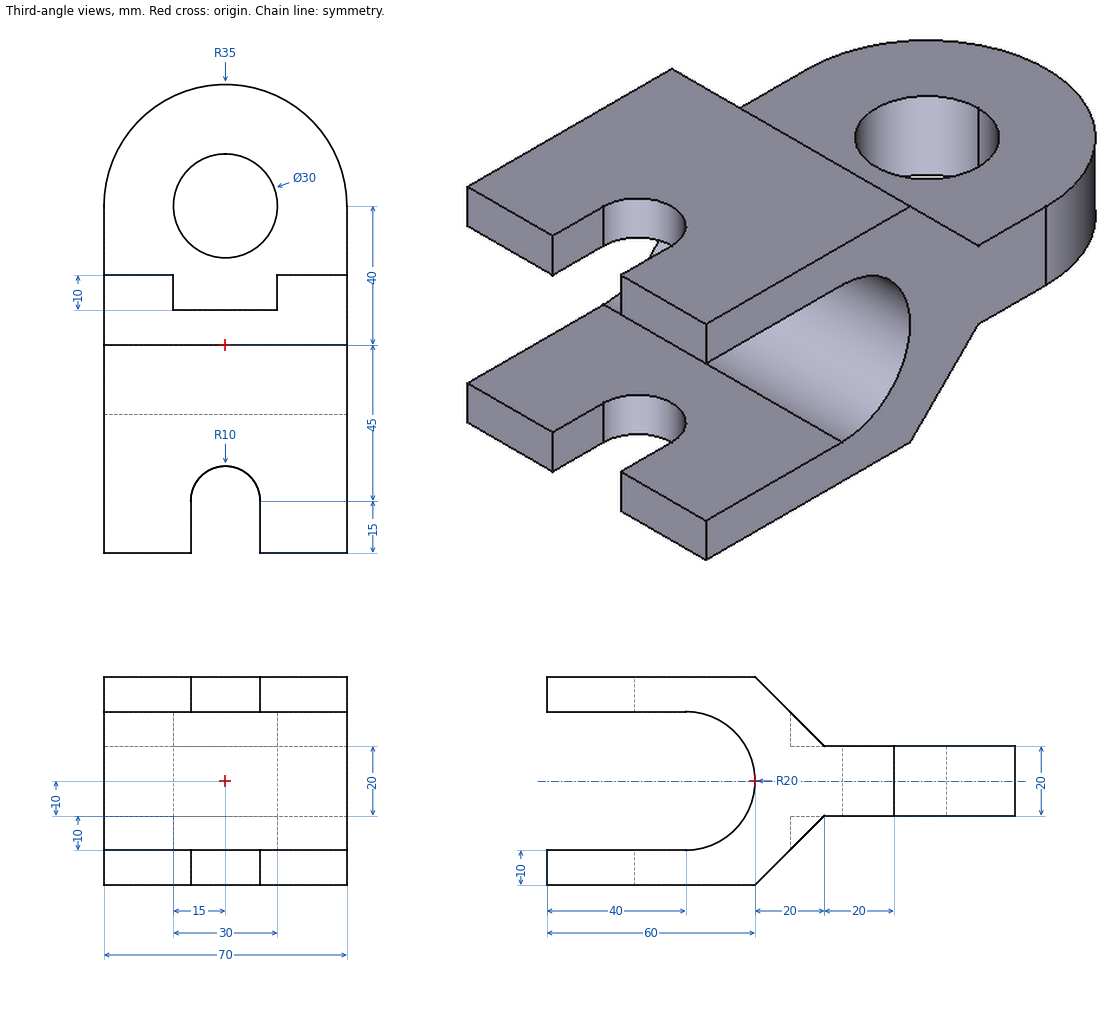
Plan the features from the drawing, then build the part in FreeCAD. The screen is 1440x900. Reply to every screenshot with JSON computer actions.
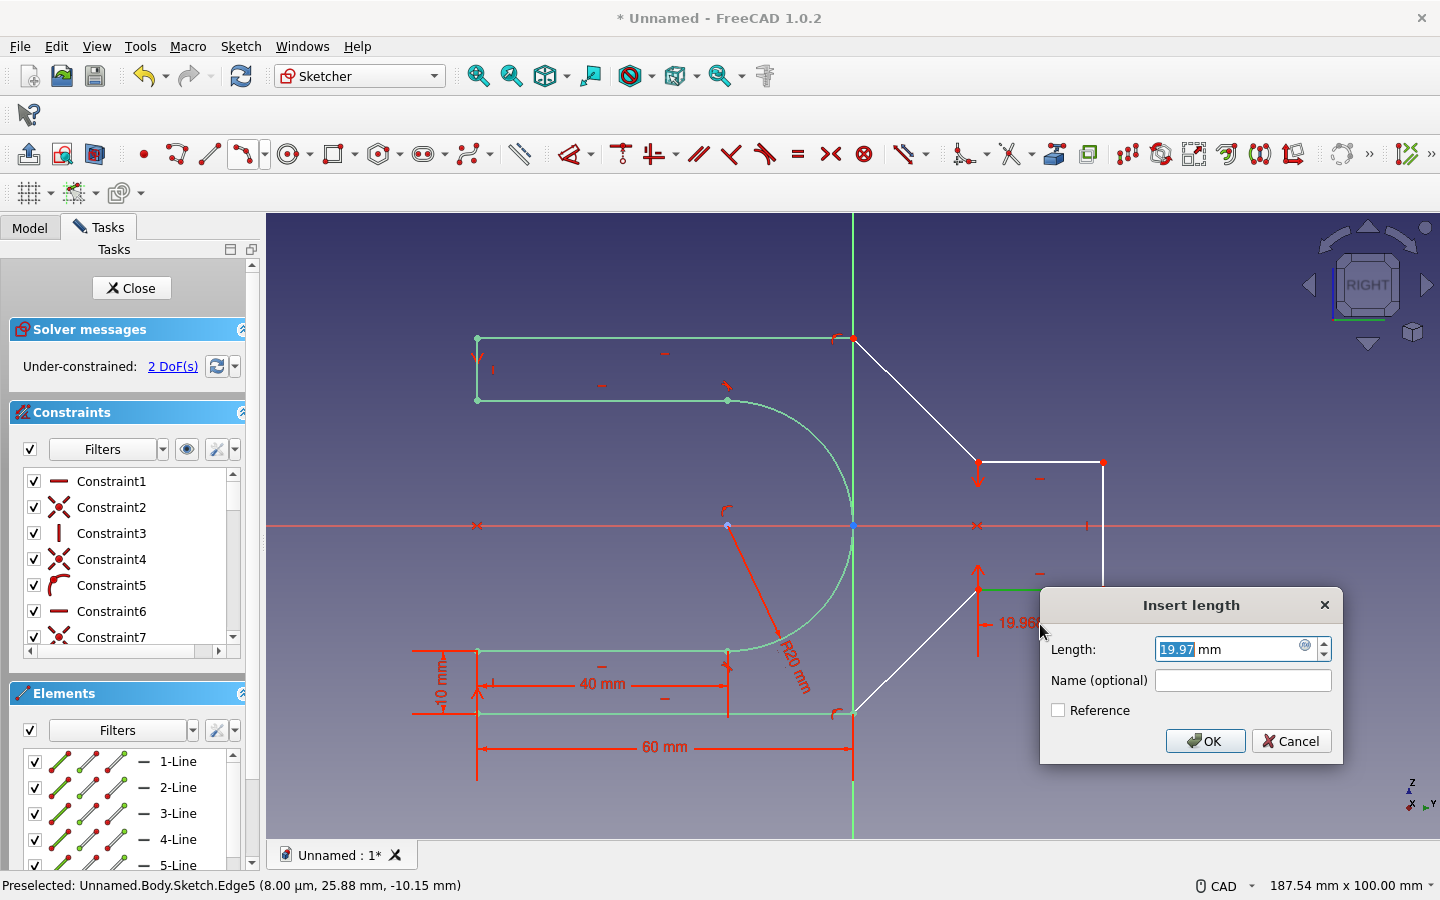
{"action": "type", "text": "20"}
{"action": "key", "text": "Return"}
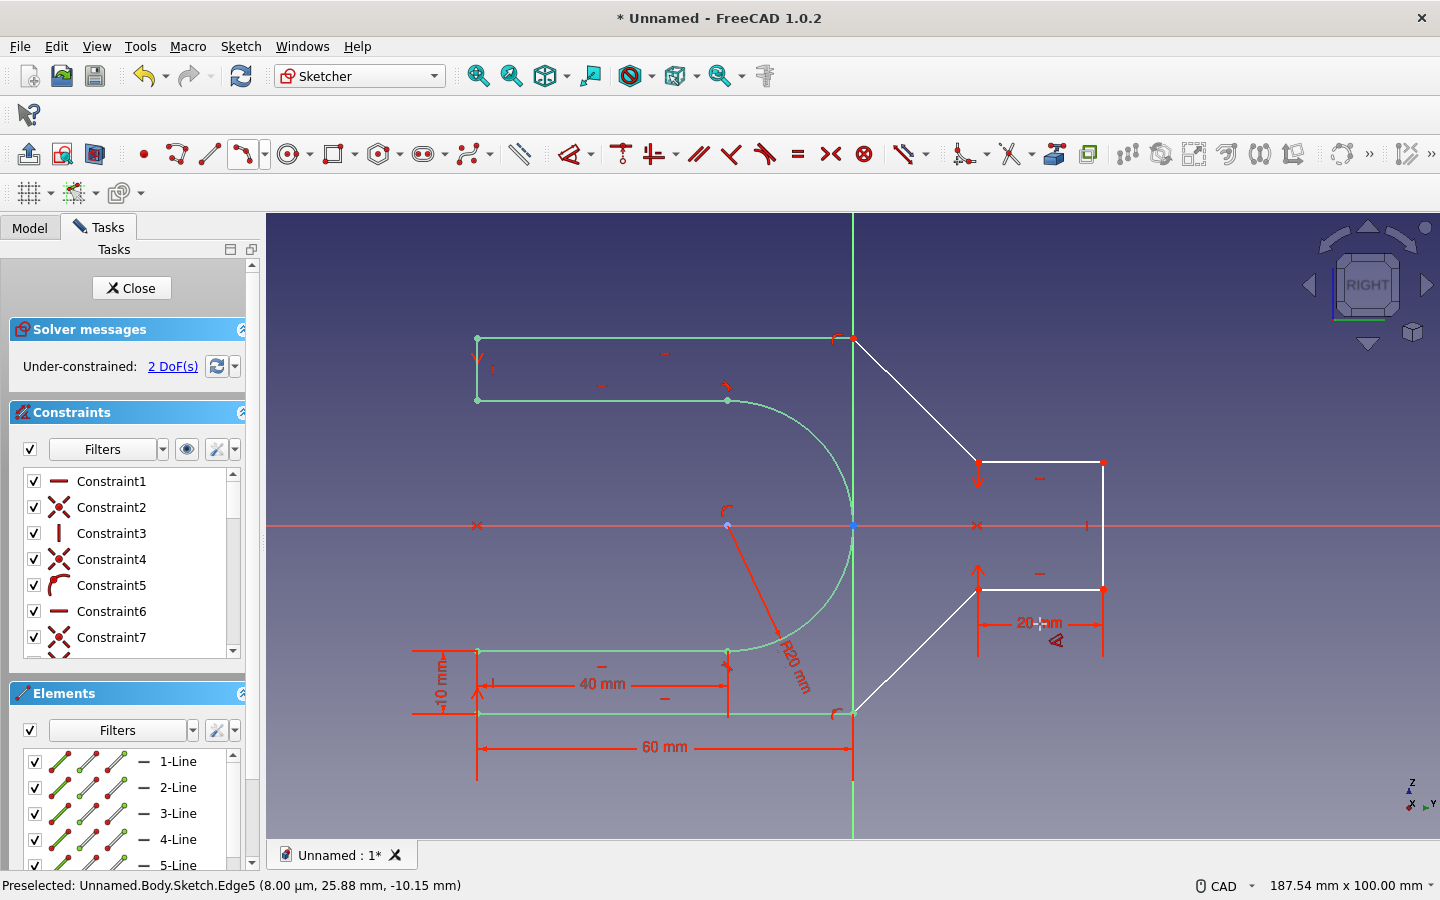
{"action": "left_click", "coordinate": [1103, 551]}
{"action": "left_click", "coordinate": [1137, 497]}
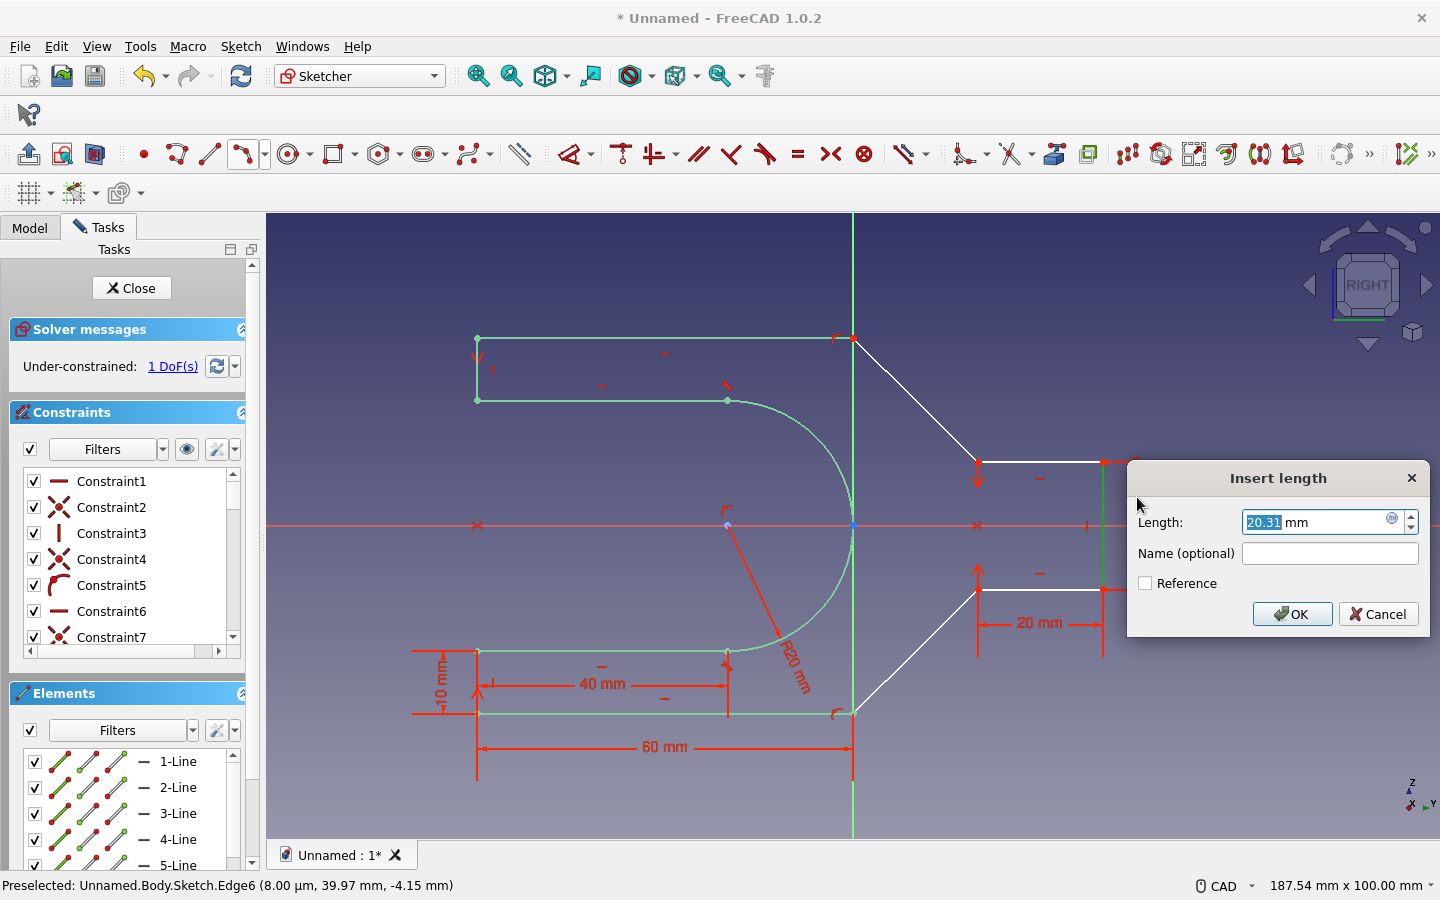
{"action": "type", "text": "20"}
{"action": "key", "text": "Return"}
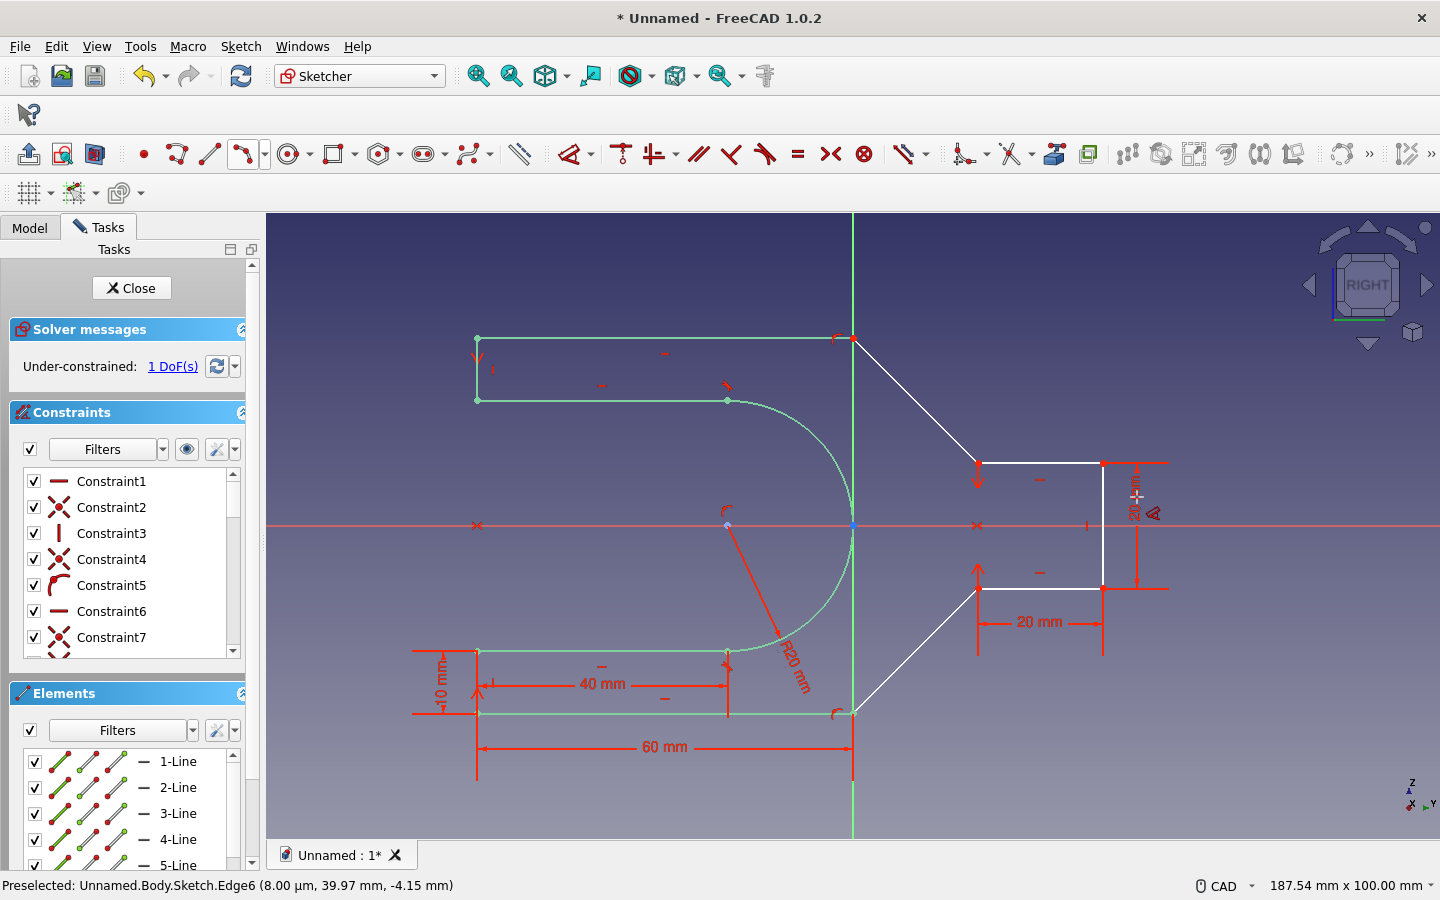
{"action": "left_click", "coordinate": [978, 589]}
{"action": "left_click", "coordinate": [915, 623]}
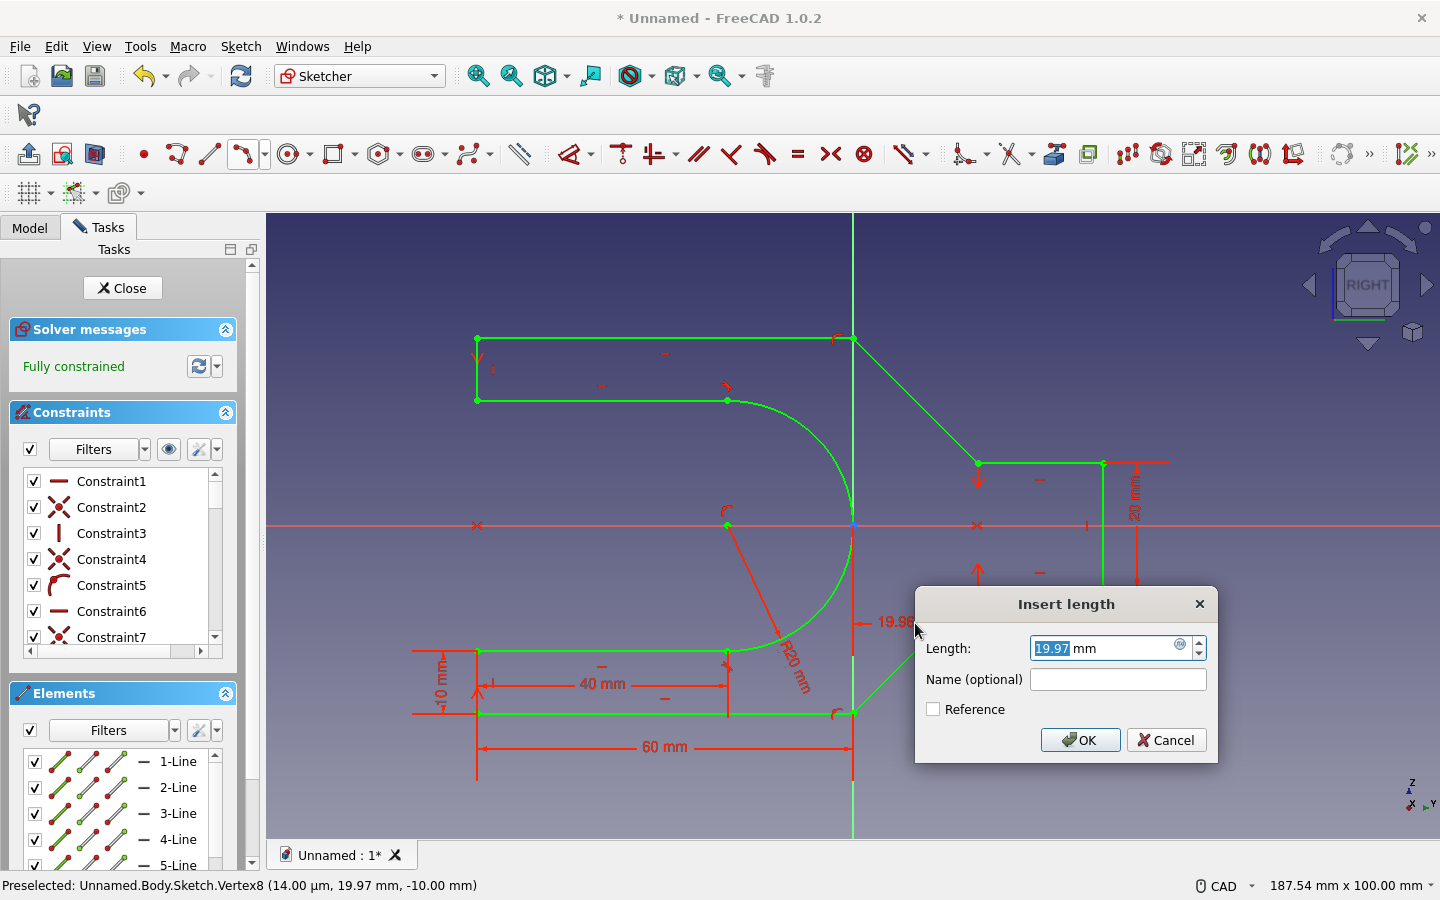
{"action": "type", "text": "20"}
{"action": "key", "text": "Return"}
{"action": "key", "text": "Escape"}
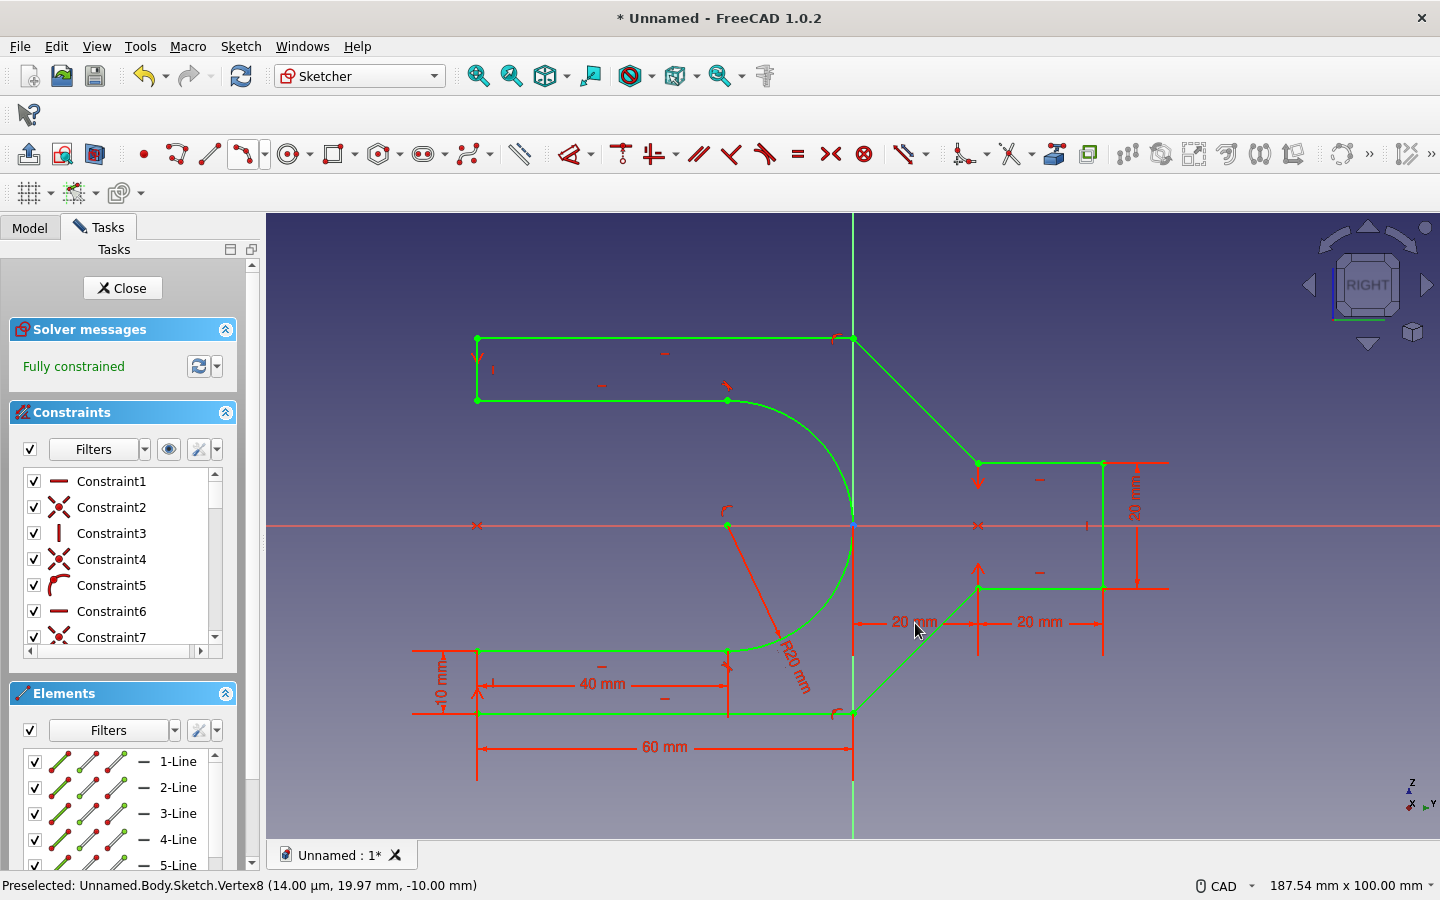
{"action": "left_click", "coordinate": [123, 288]}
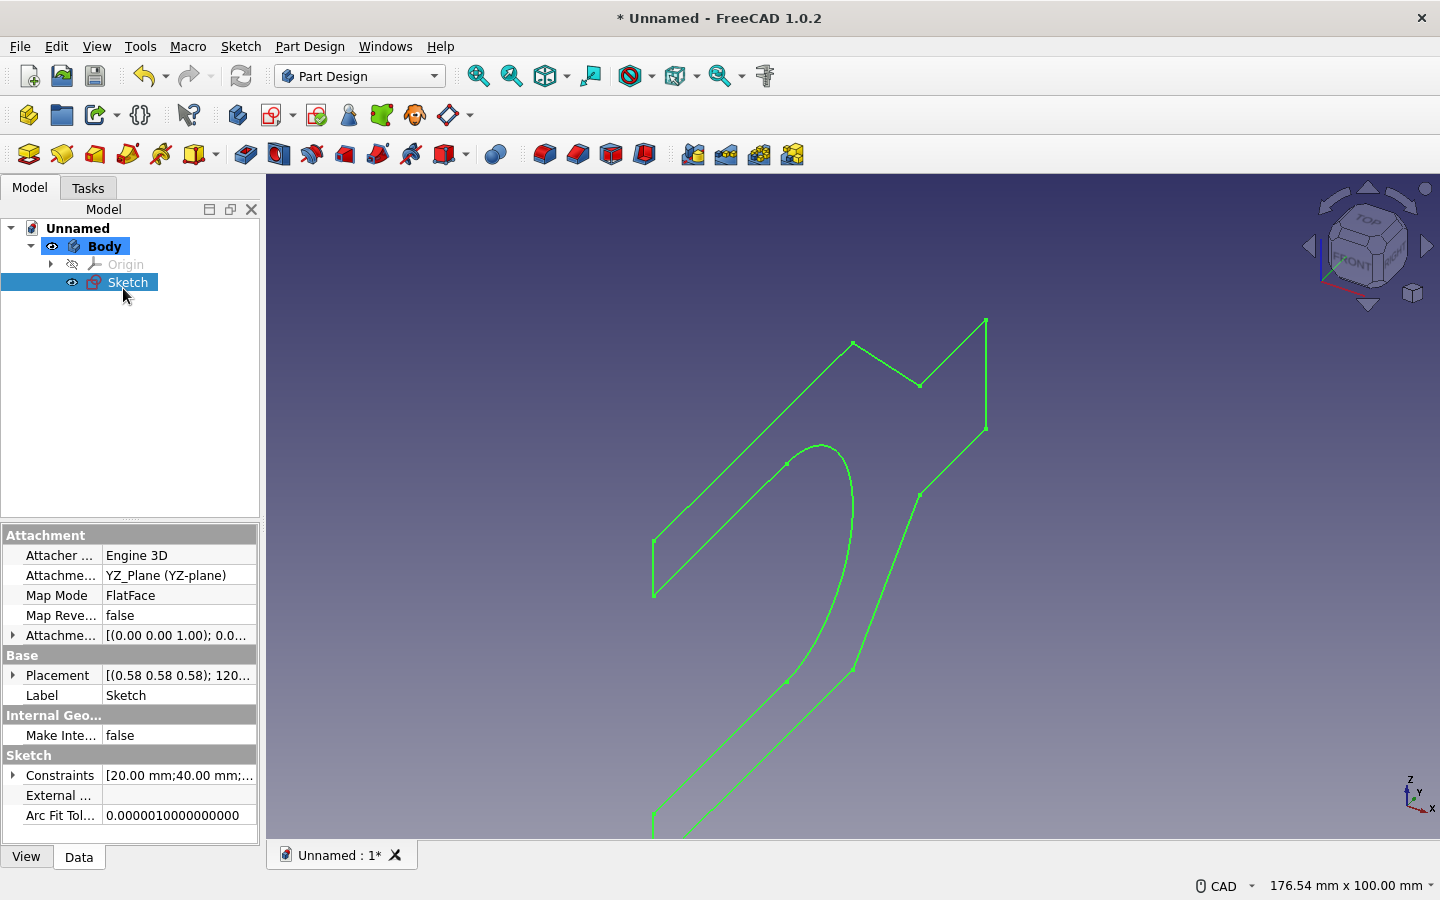
{"action": "left_click", "coordinate": [29, 154]}